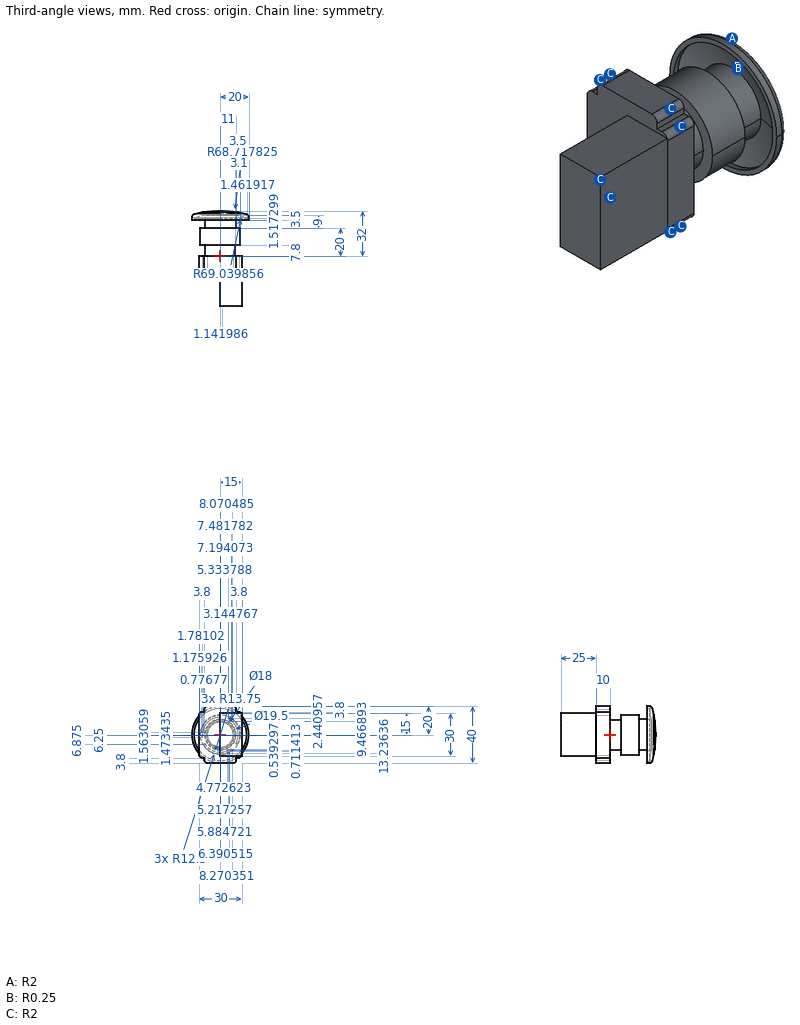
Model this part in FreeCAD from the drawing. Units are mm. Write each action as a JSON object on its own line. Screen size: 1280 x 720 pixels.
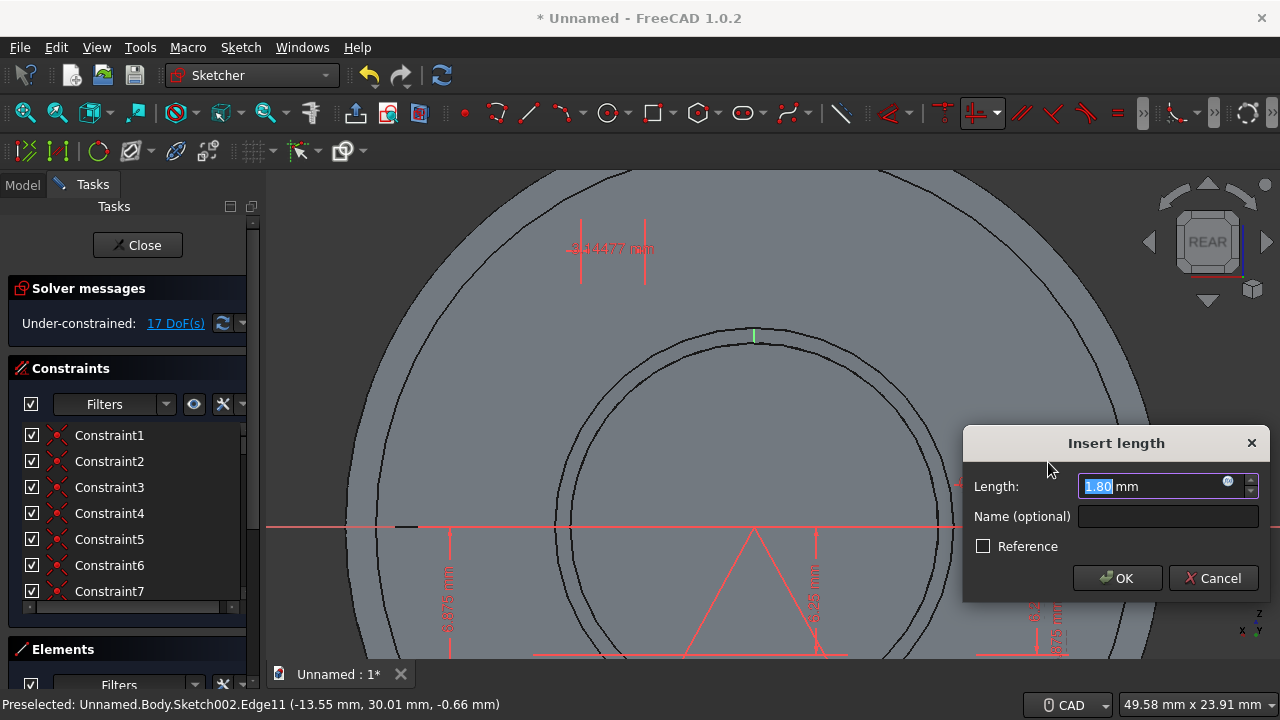
{"action": "type", "text": "1.78102"}
{"action": "key", "text": "Return"}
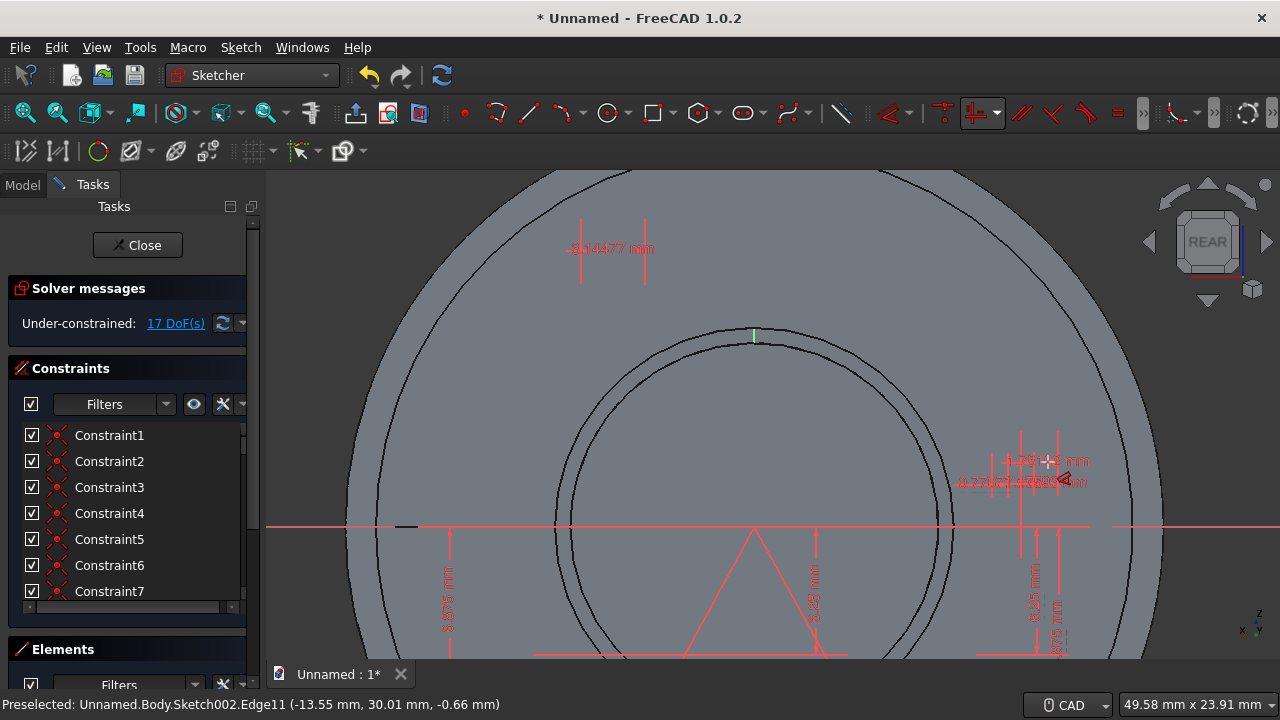
{"action": "scroll", "coordinate": [627, 284], "scroll_direction": "down", "scroll_amount": 3}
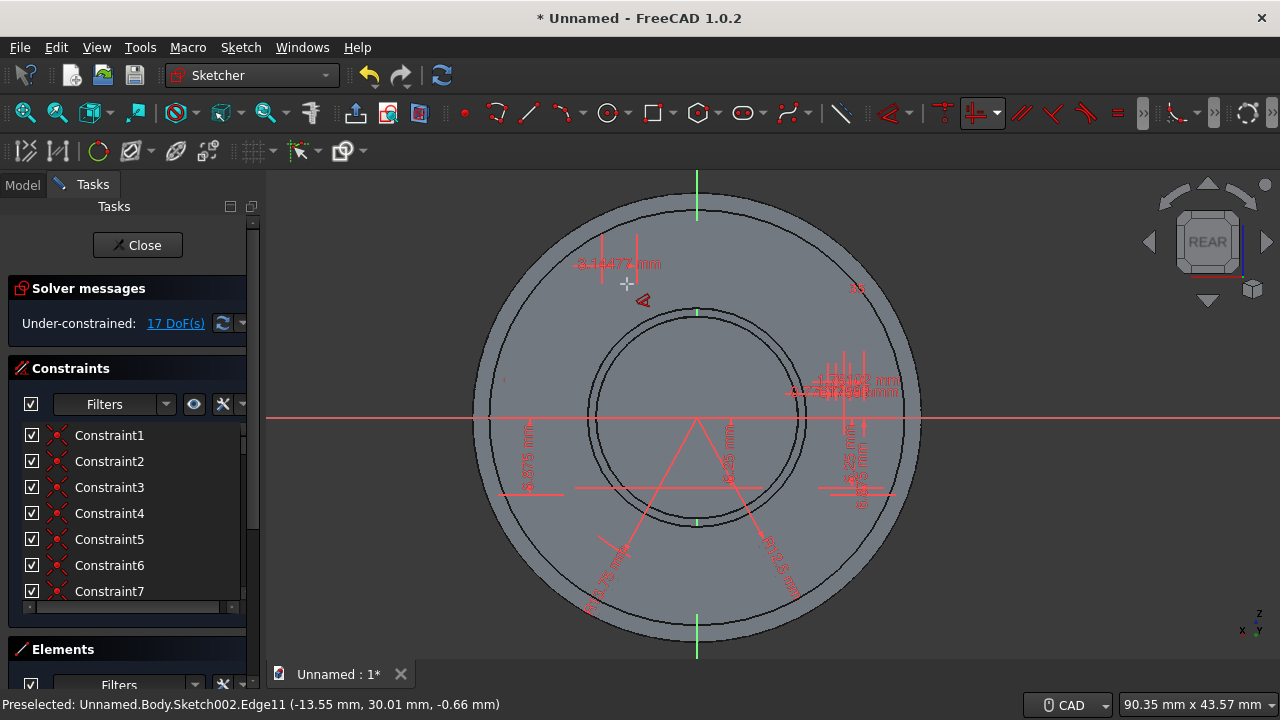
{"action": "scroll", "coordinate": [638, 545], "scroll_direction": "up", "scroll_amount": 2}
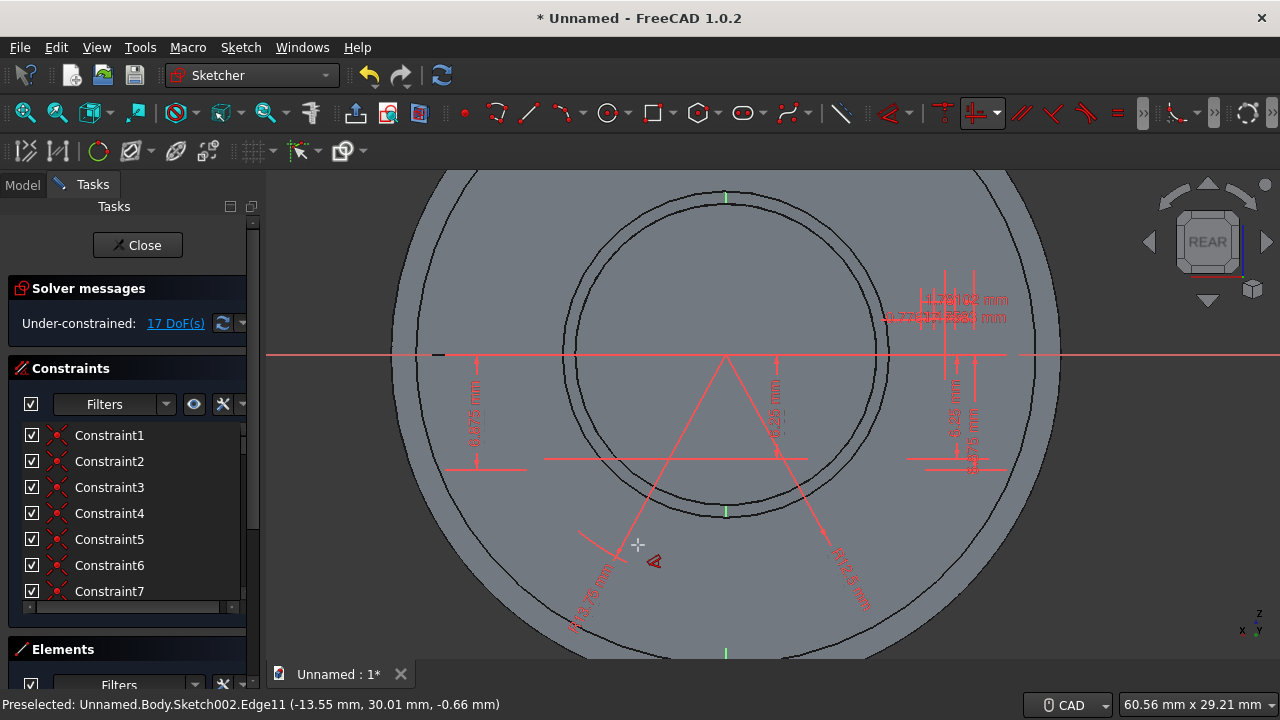
{"action": "left_click", "coordinate": [638, 545]}
{"action": "left_click", "coordinate": [682, 321]}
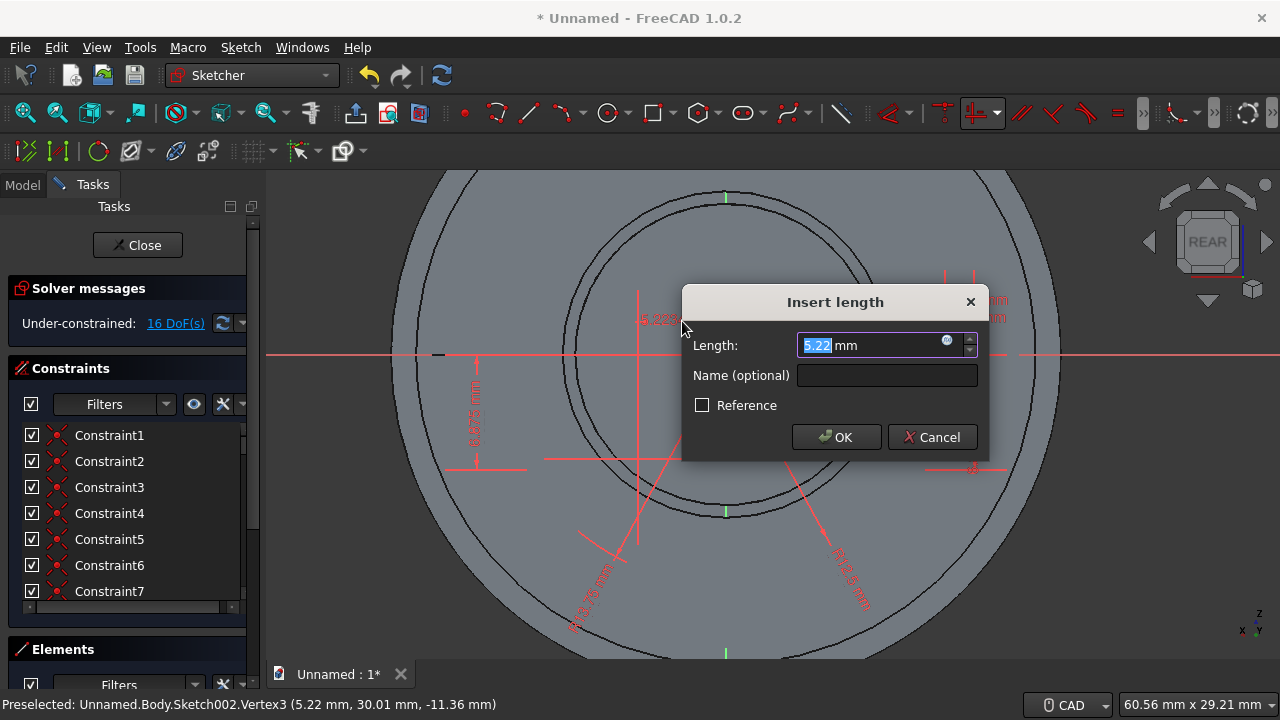
{"action": "type", "text": "5.217257"}
{"action": "key", "text": "Return"}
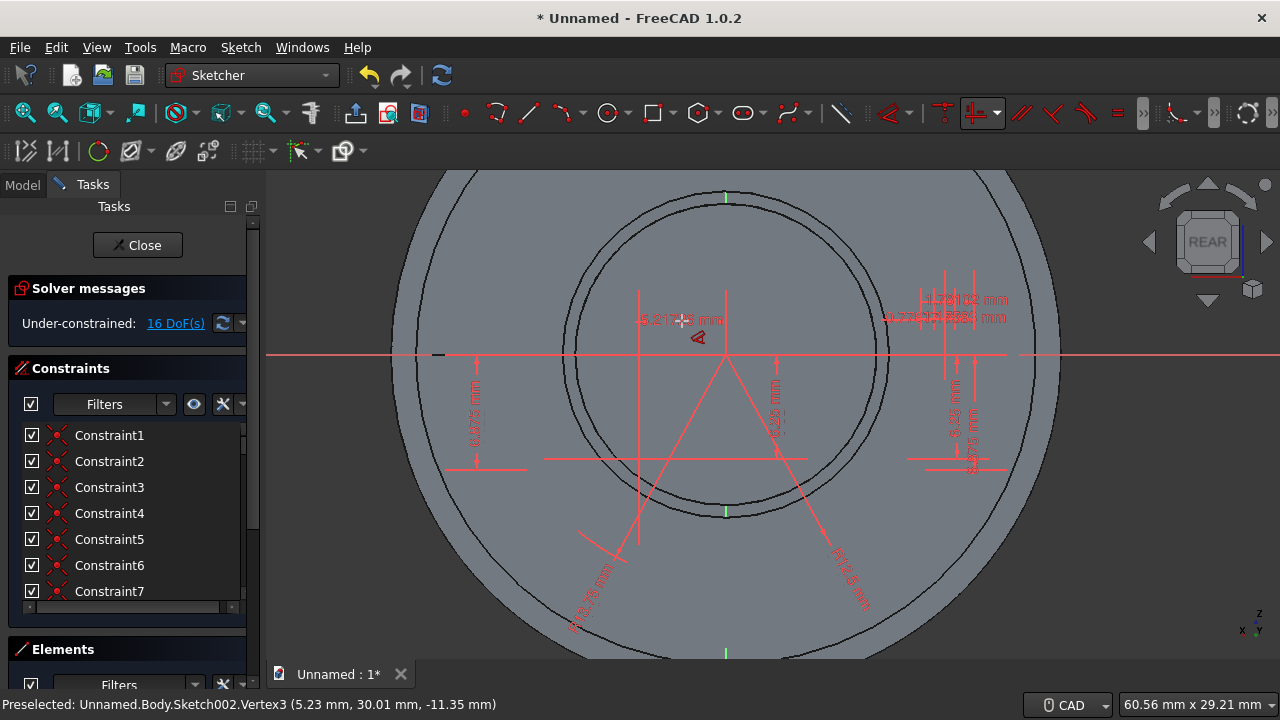
{"action": "left_click", "coordinate": [646, 533]}
{"action": "left_click", "coordinate": [668, 591]}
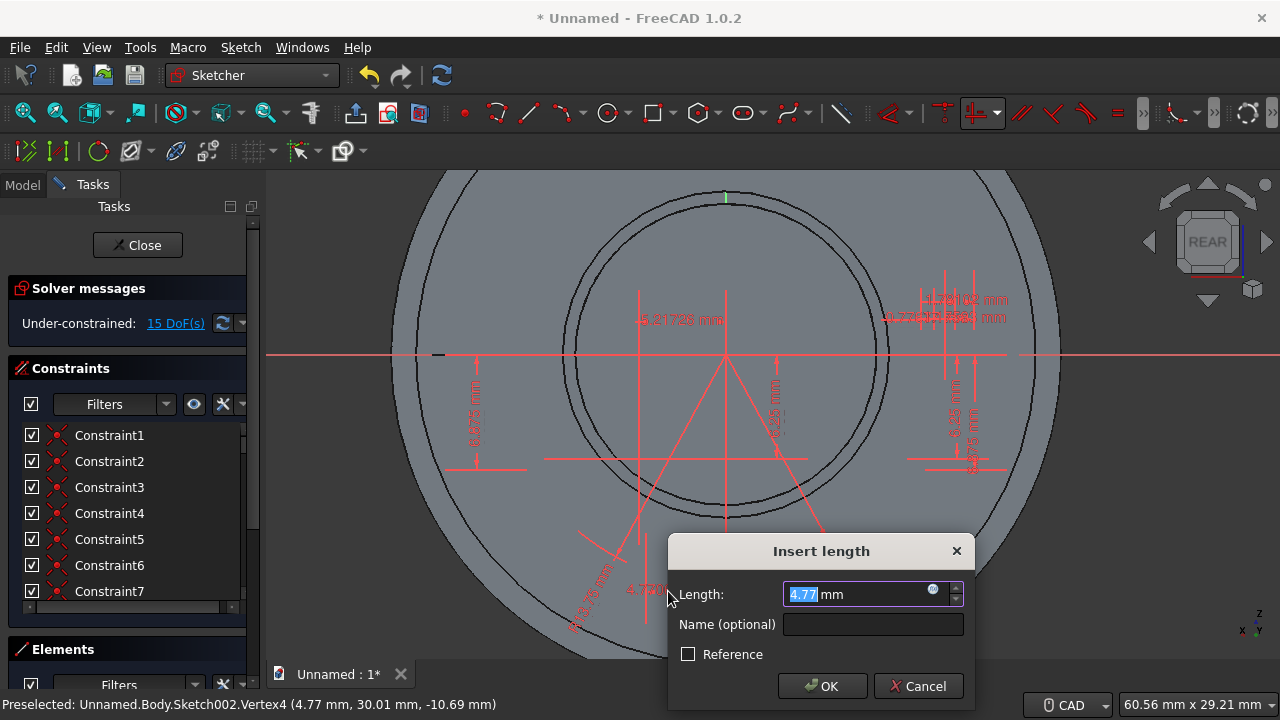
{"action": "type", "text": "4.772623"}
{"action": "key", "text": "Return"}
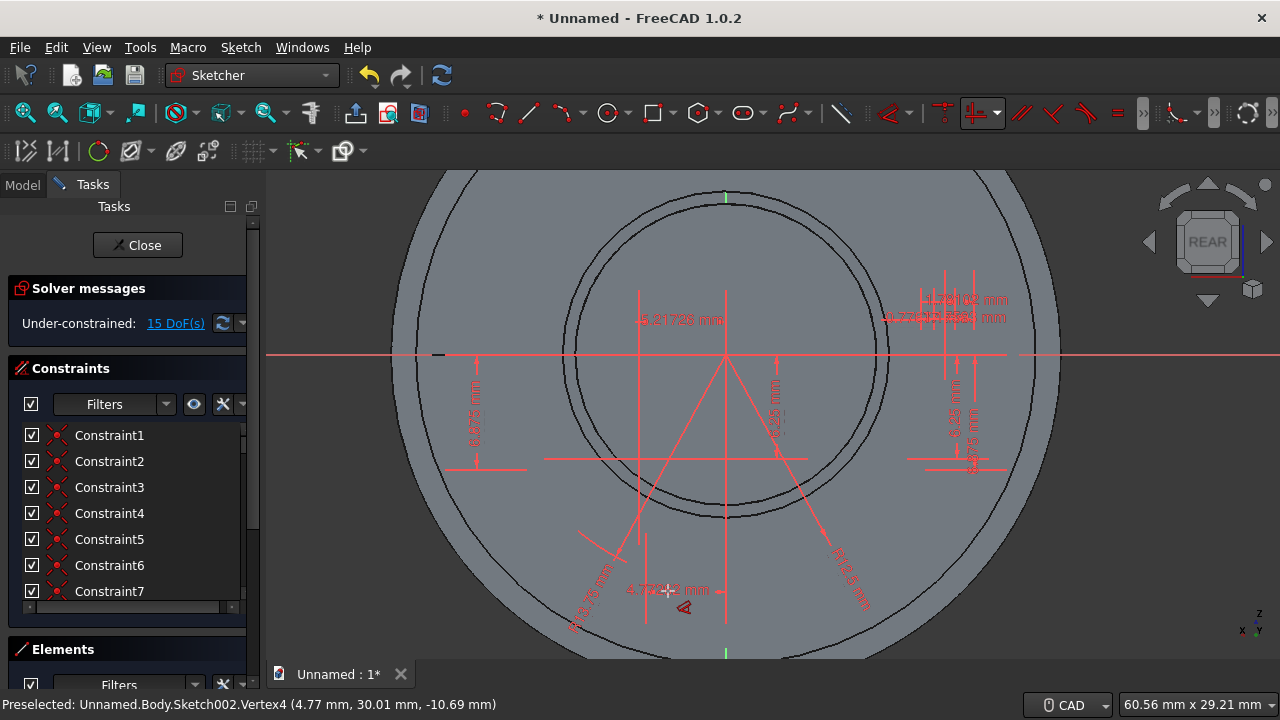
{"action": "left_click", "coordinate": [587, 524]}
{"action": "left_click", "coordinate": [608, 321]}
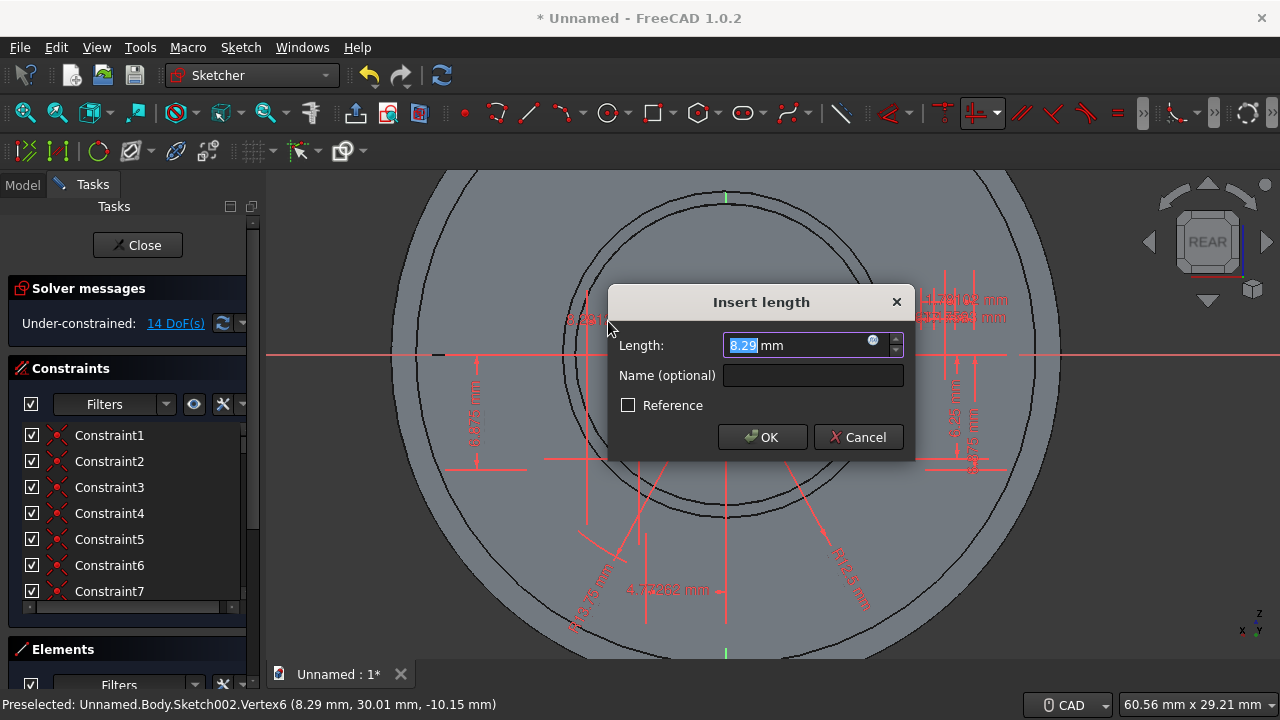
{"action": "type", "text": "8.270351"}
{"action": "key", "text": "Return"}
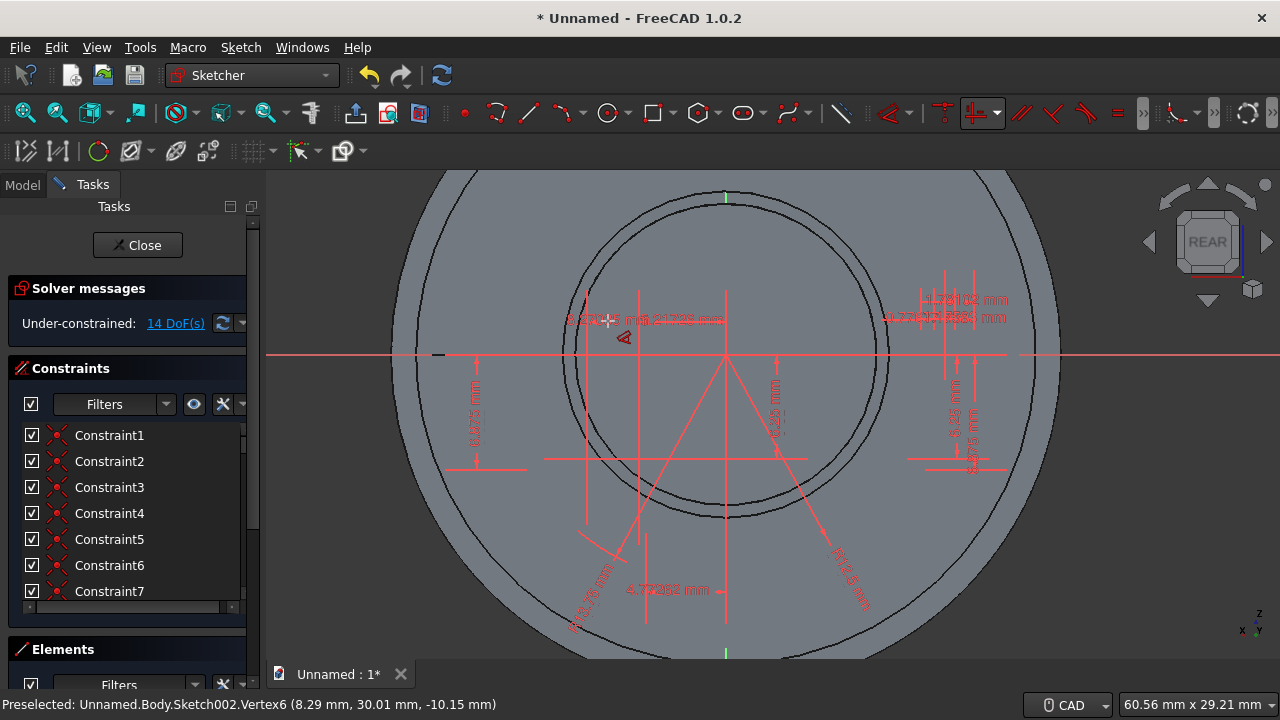
{"action": "left_click", "coordinate": [619, 577]}
{"action": "left_click", "coordinate": [672, 297]}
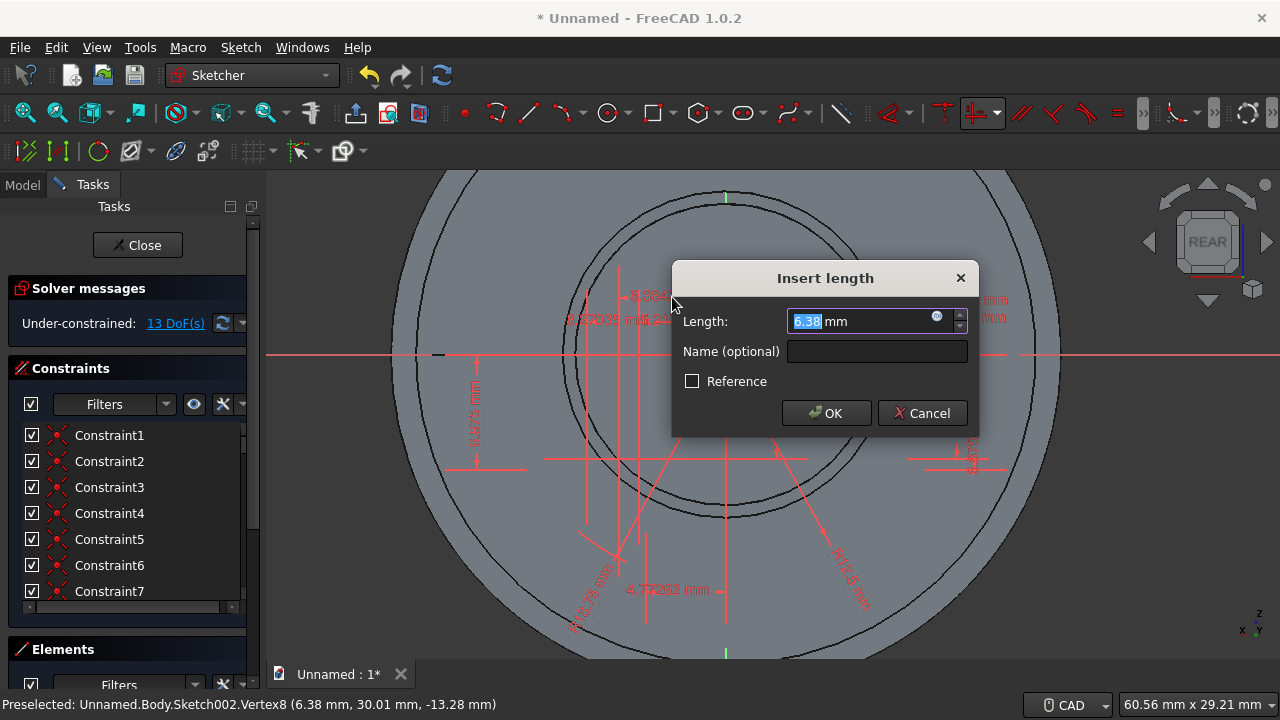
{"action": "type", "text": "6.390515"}
{"action": "key", "text": "Return"}